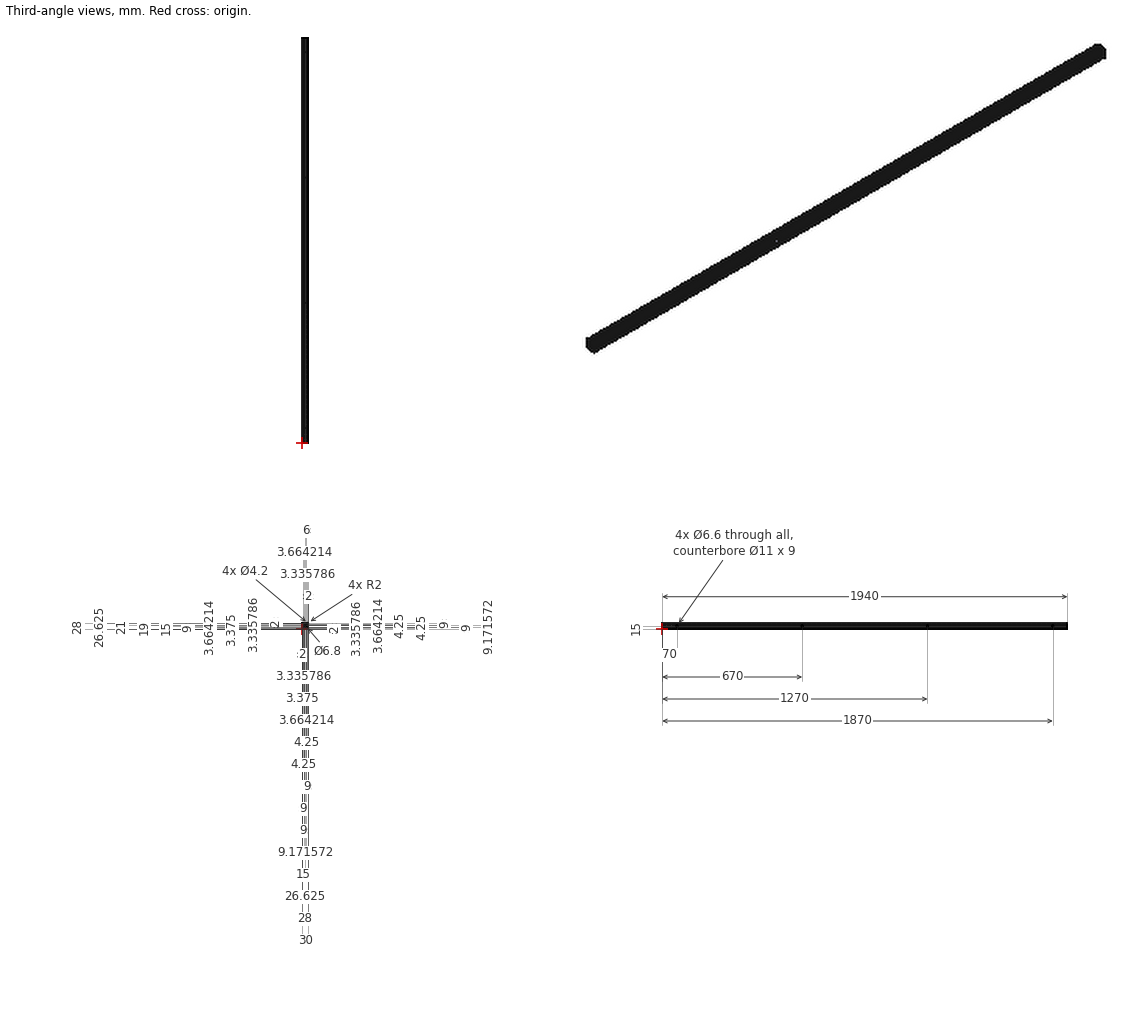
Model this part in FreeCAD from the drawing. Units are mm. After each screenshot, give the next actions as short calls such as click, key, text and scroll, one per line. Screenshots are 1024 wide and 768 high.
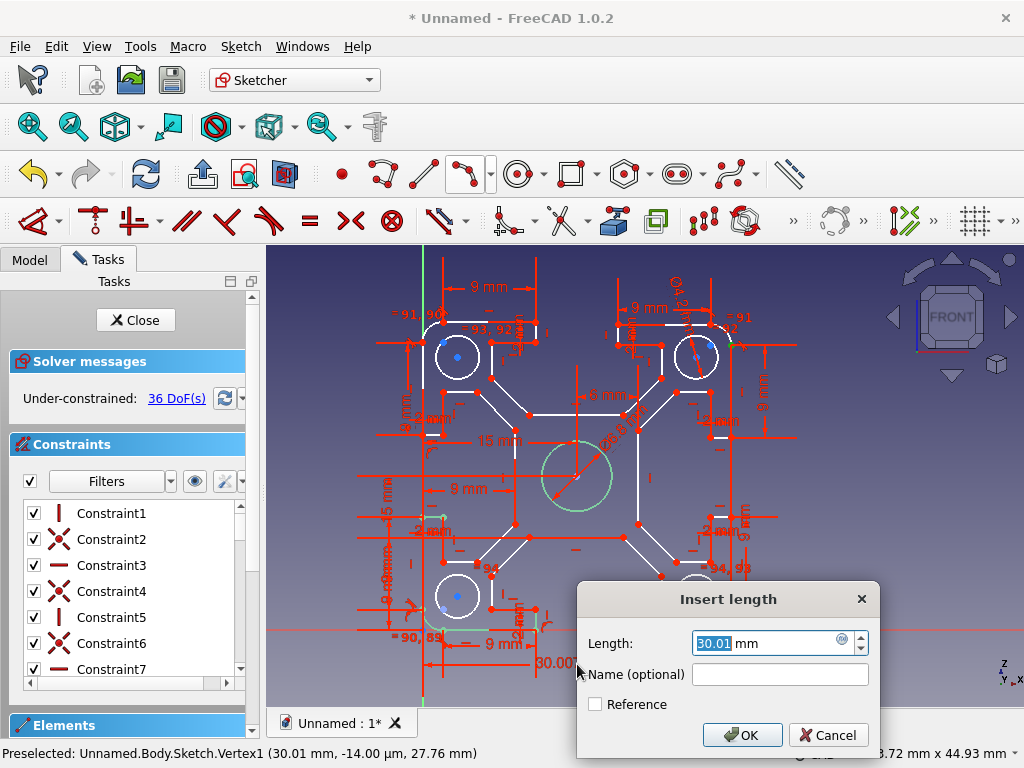
text(30)
key(Return)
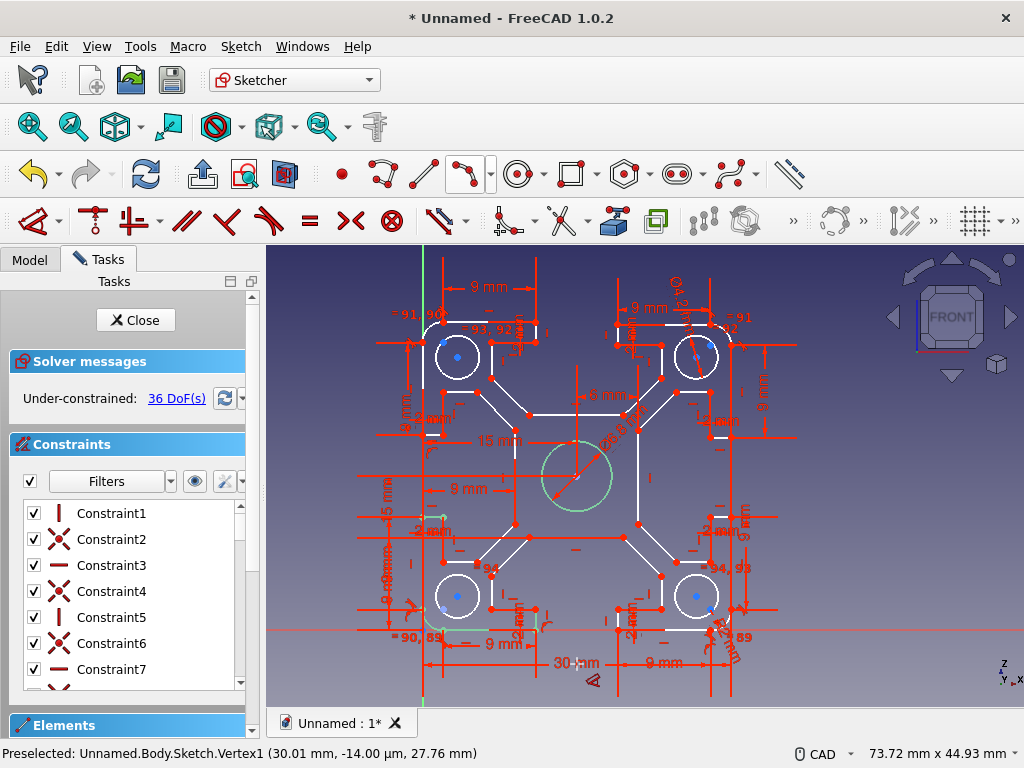
click(731, 345)
click(765, 488)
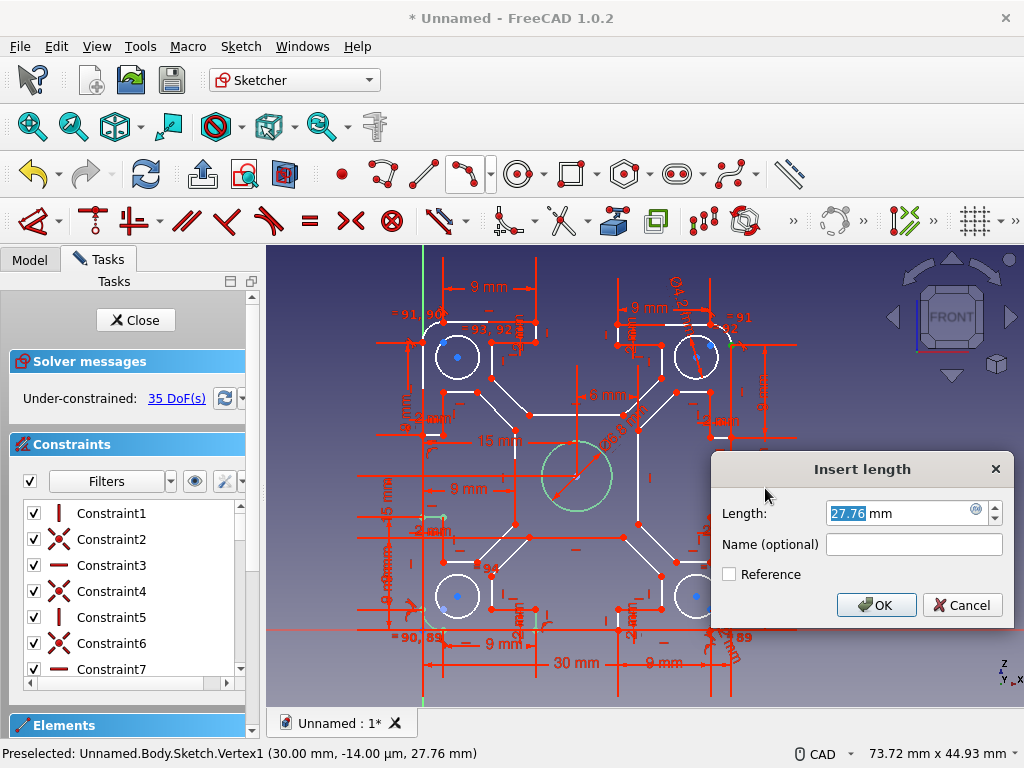
text(28)
key(Return)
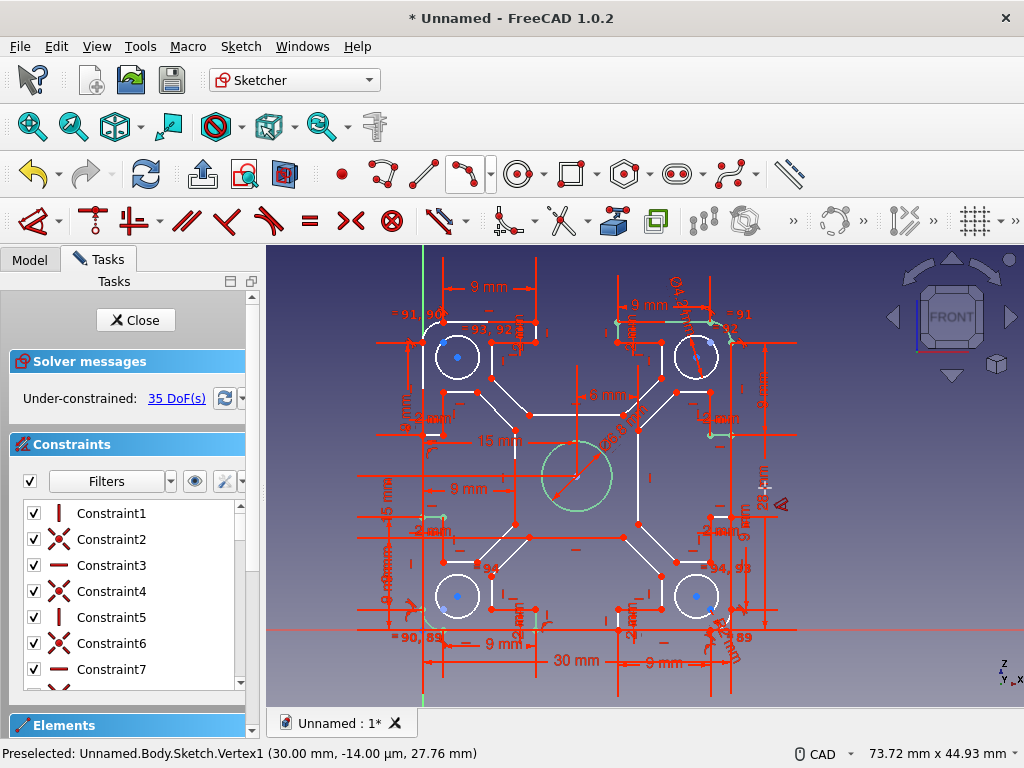
click(711, 562)
click(667, 504)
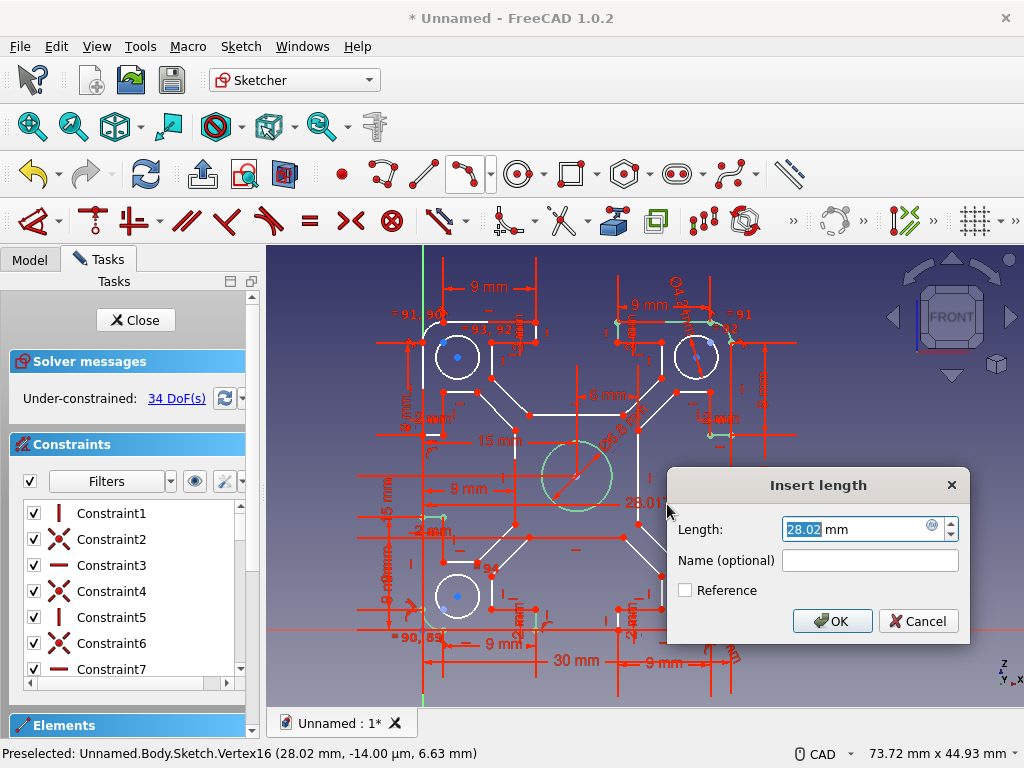
text(28)
key(Return)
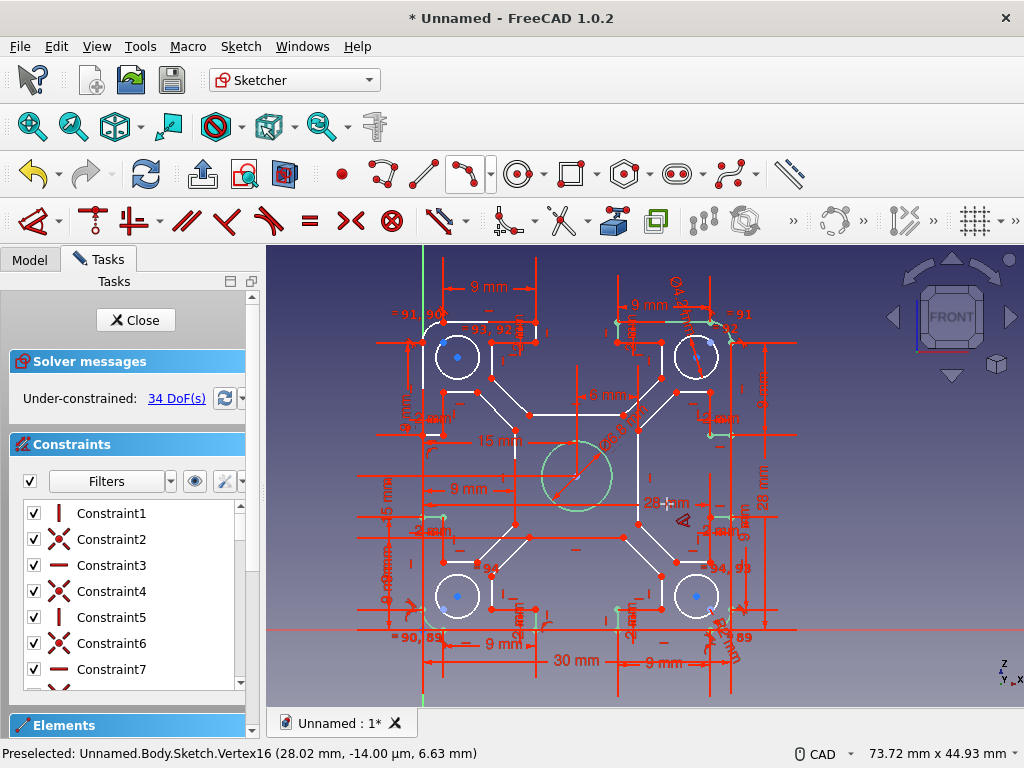
click(443, 435)
click(389, 464)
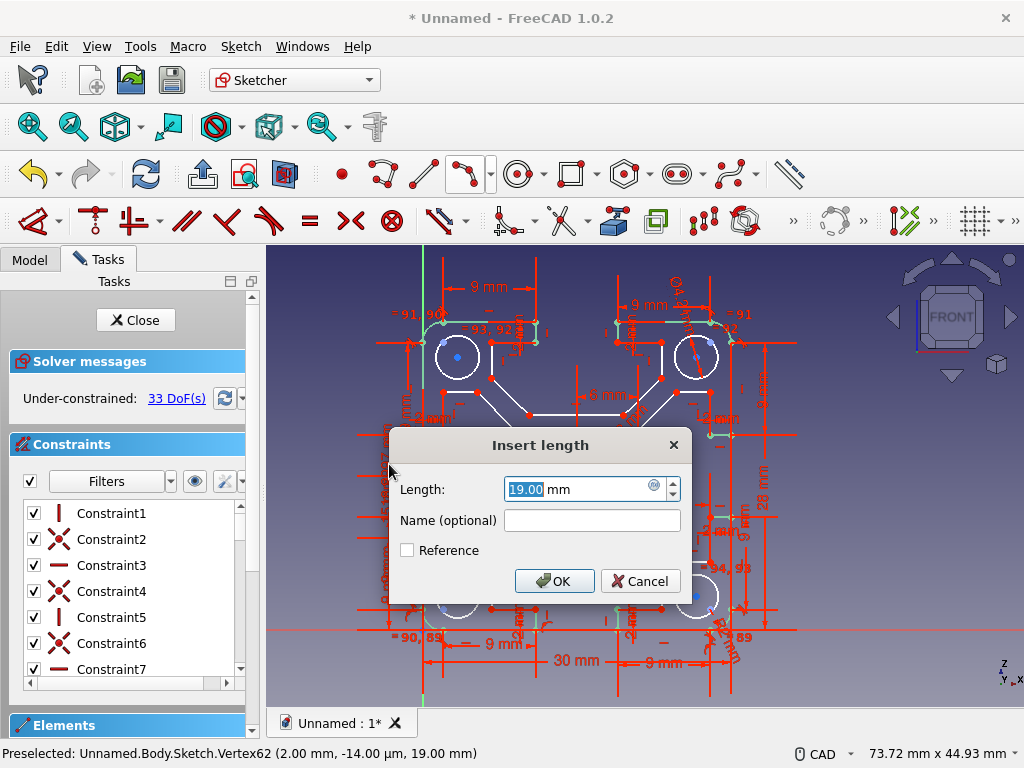
text(19)
key(Return)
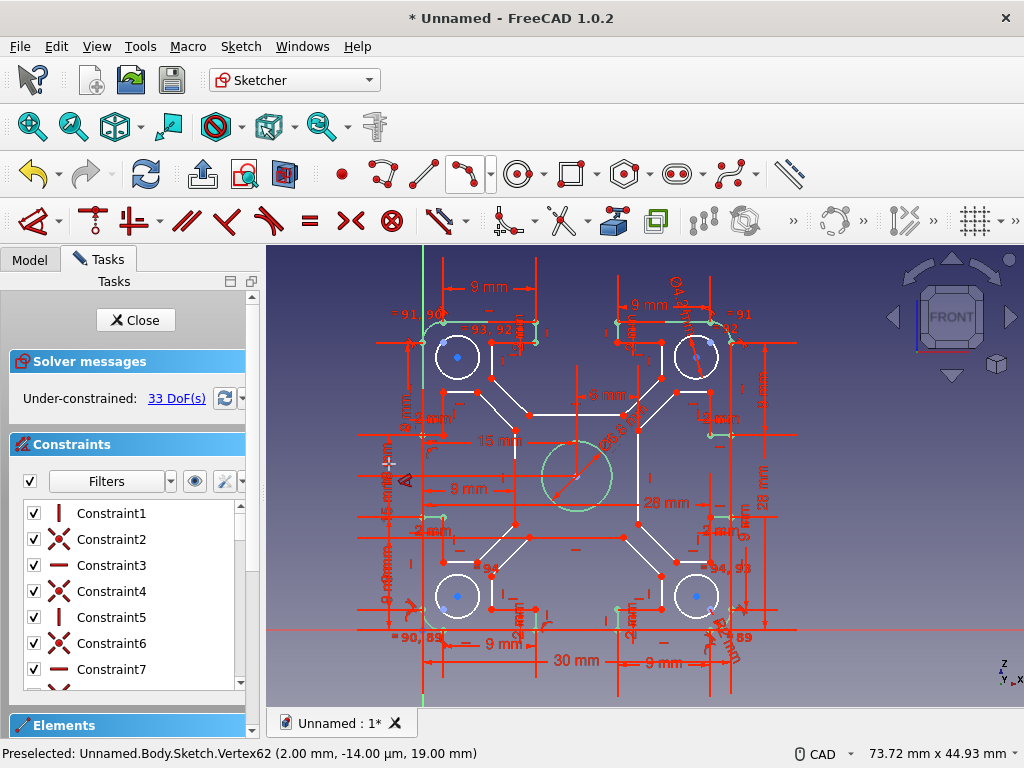
click(530, 415)
click(564, 523)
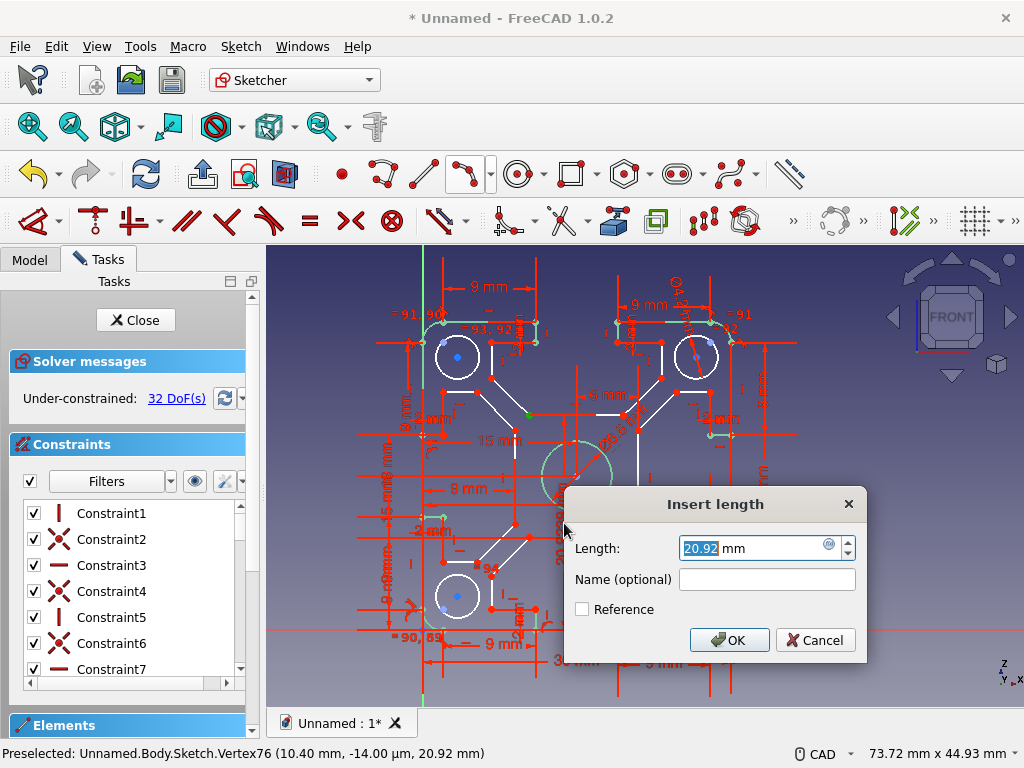
text(21)
key(Return)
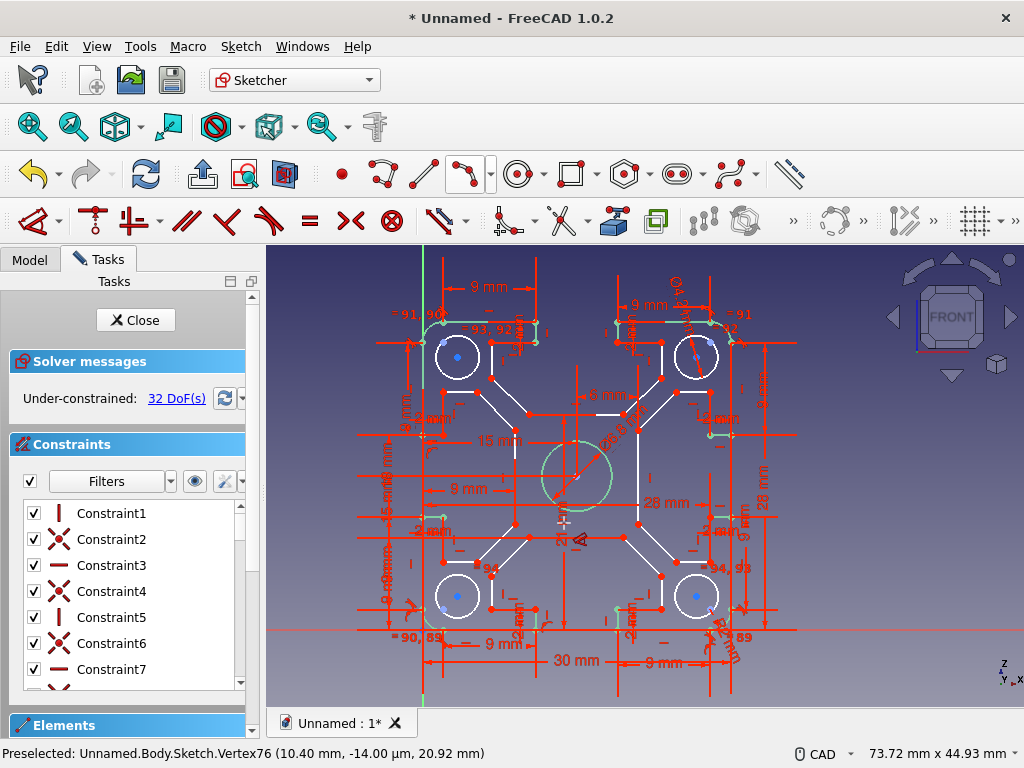
click(710, 422)
click(792, 414)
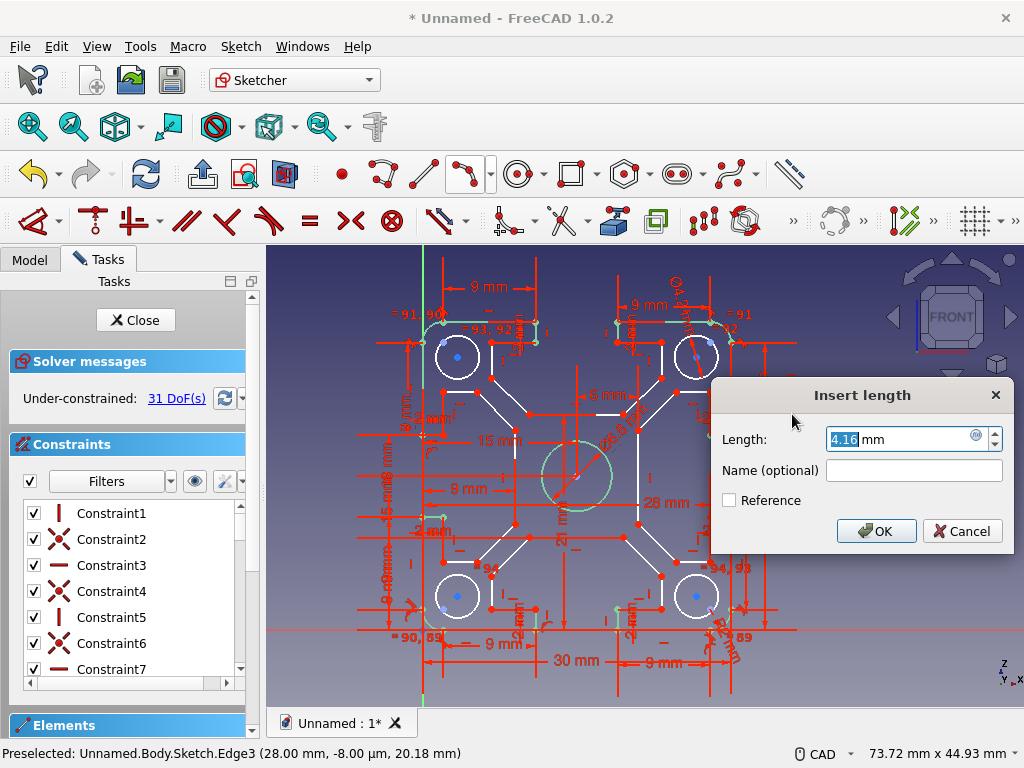
text(4.25)
key(Return)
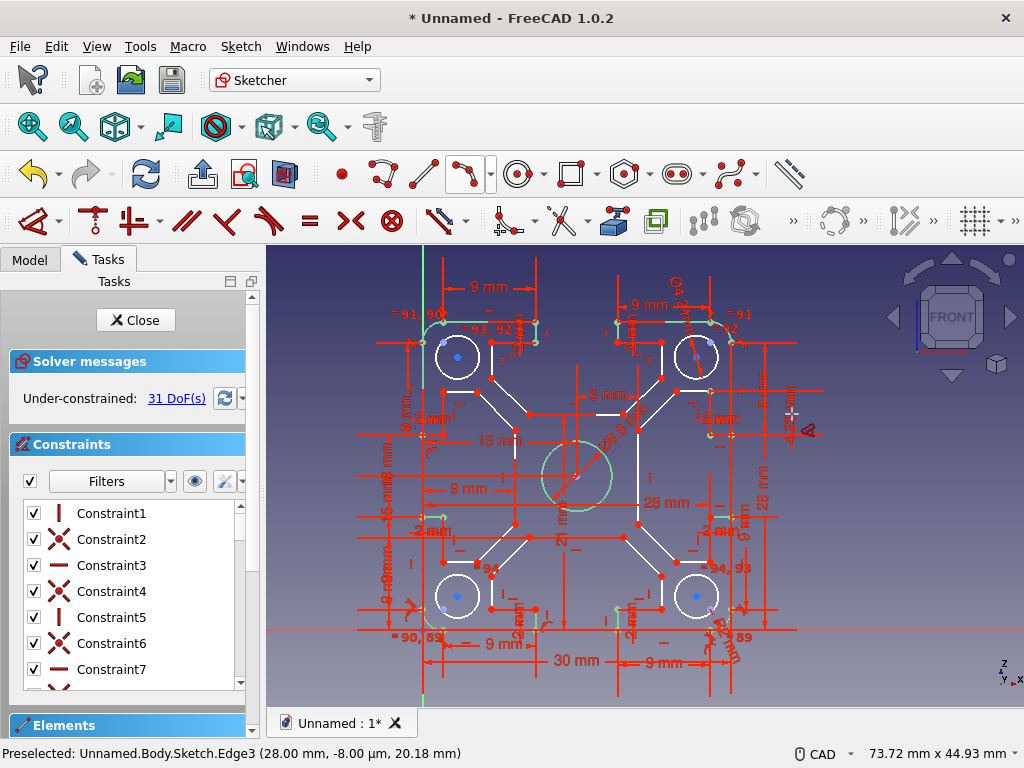
click(710, 549)
click(744, 556)